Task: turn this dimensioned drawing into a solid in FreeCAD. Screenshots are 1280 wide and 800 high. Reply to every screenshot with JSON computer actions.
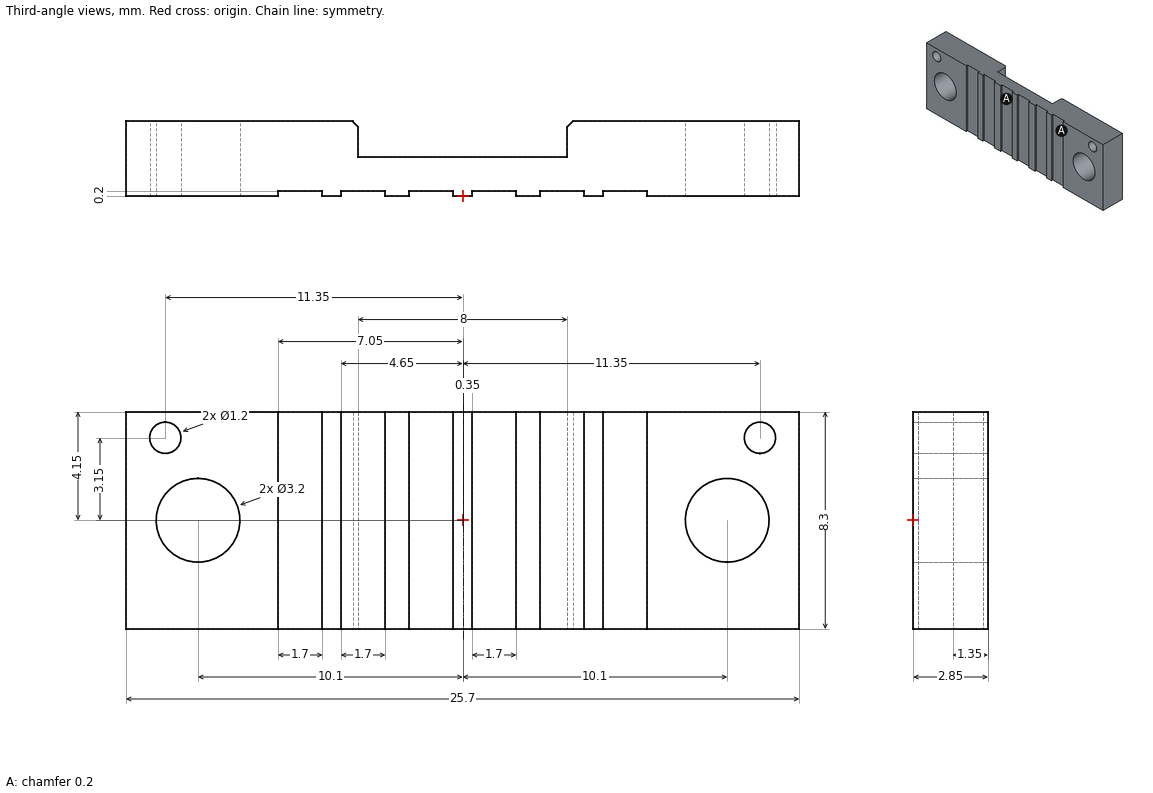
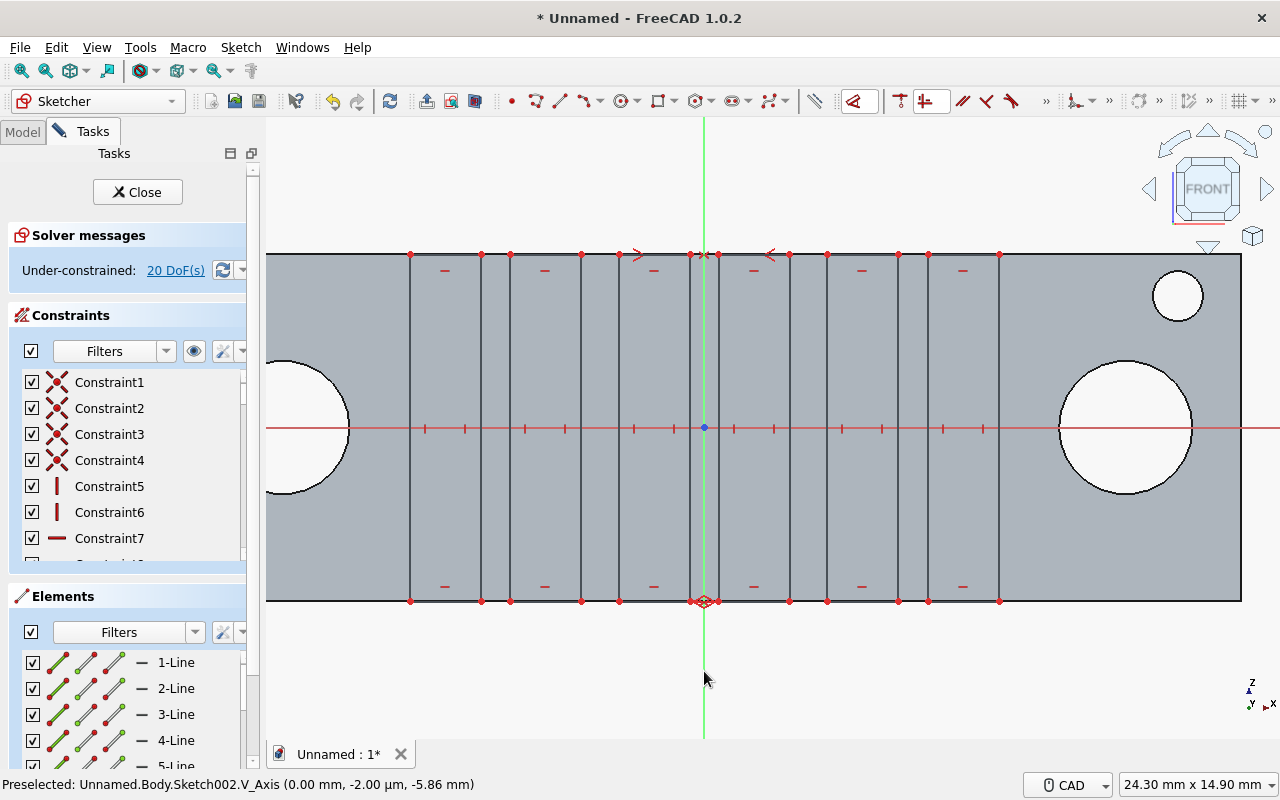
{"action": "left_click", "coordinate": [581, 255]}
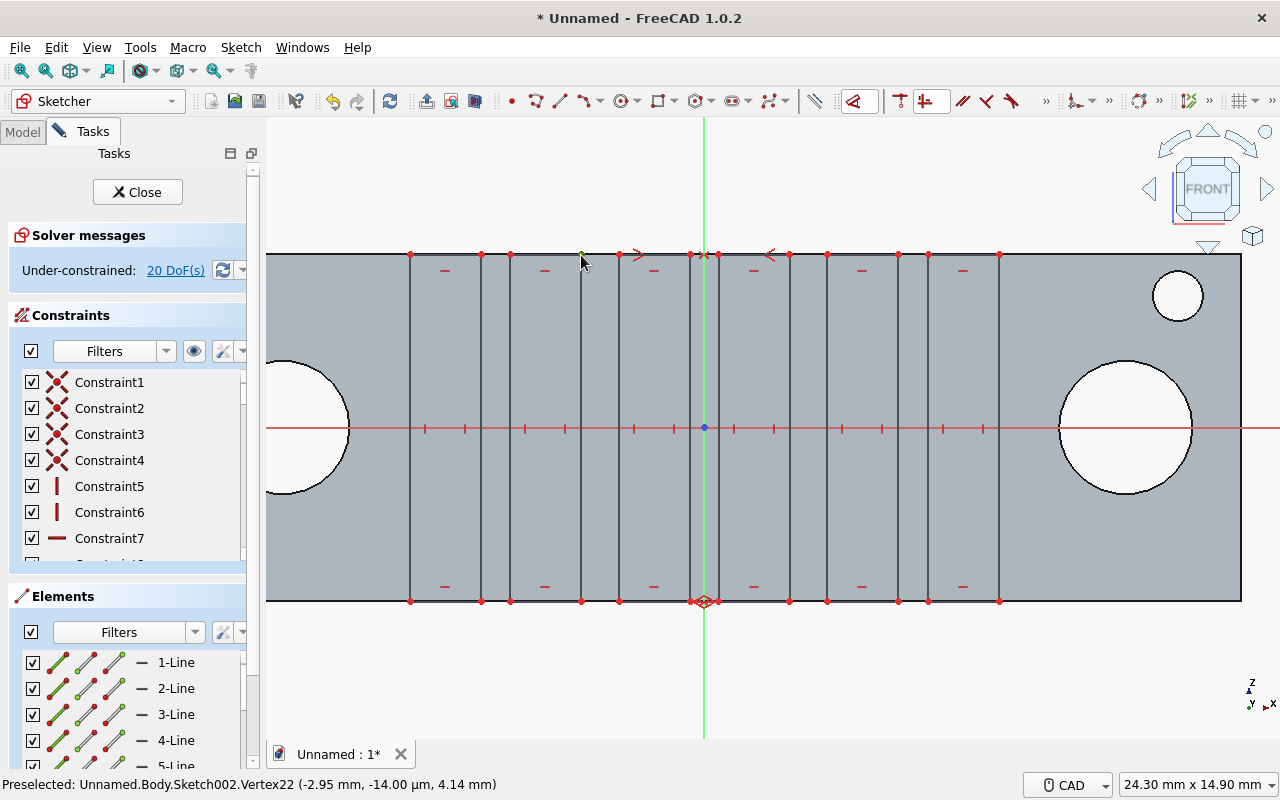
{"action": "left_click", "coordinate": [827, 255]}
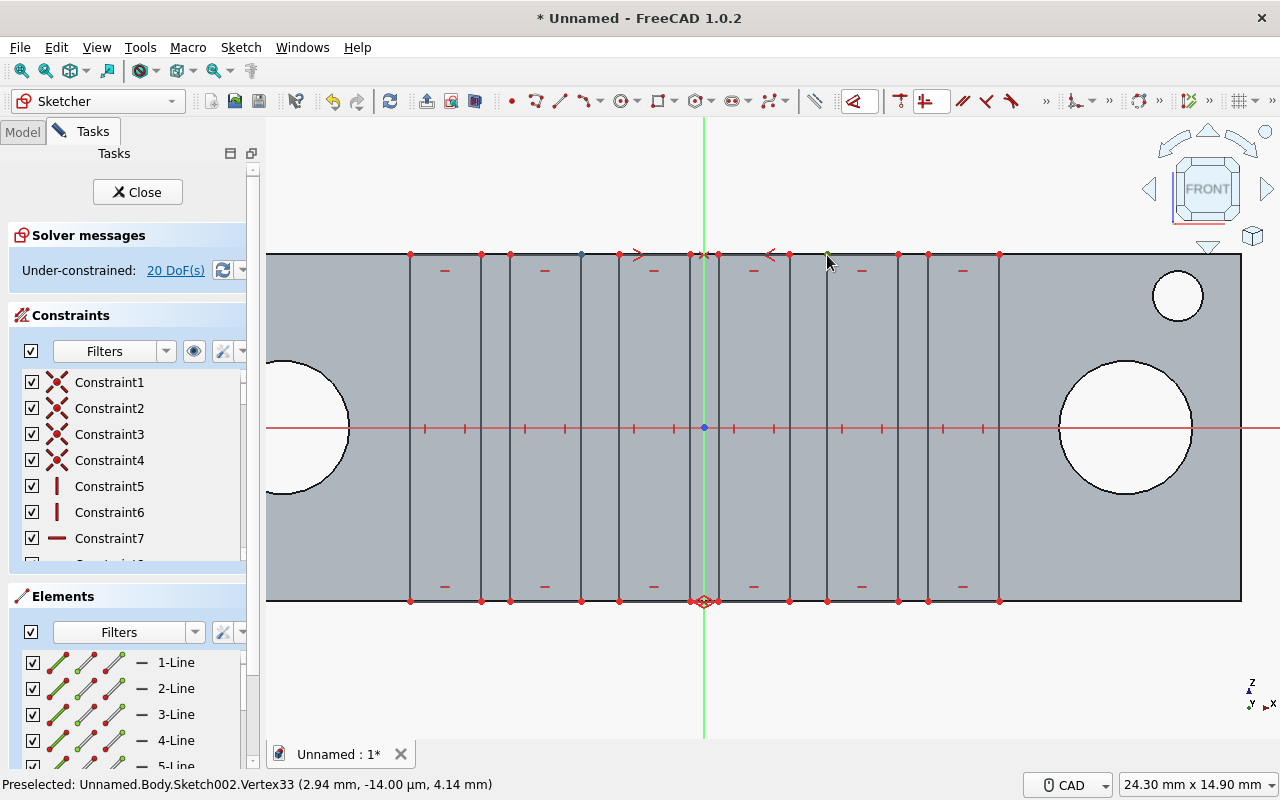
{"action": "left_click", "coordinate": [704, 671]}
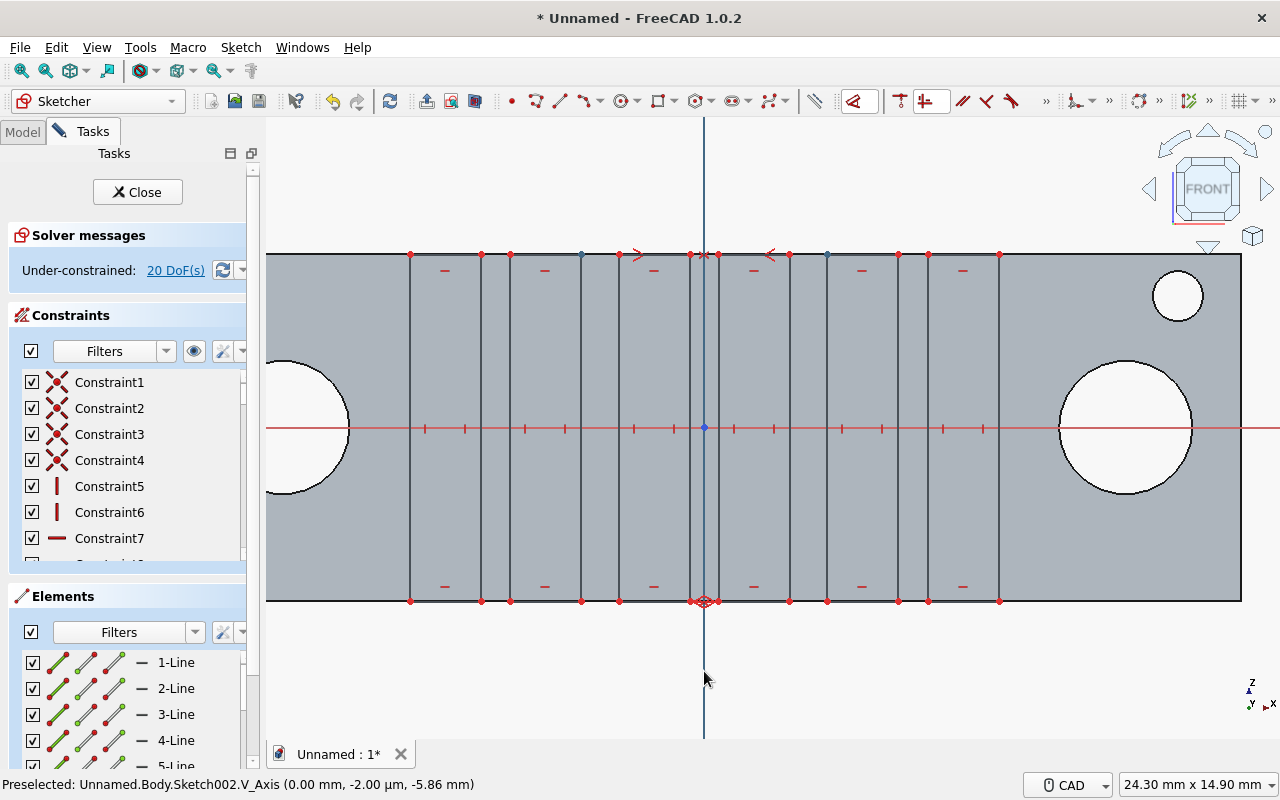
{"action": "key", "text": "s"}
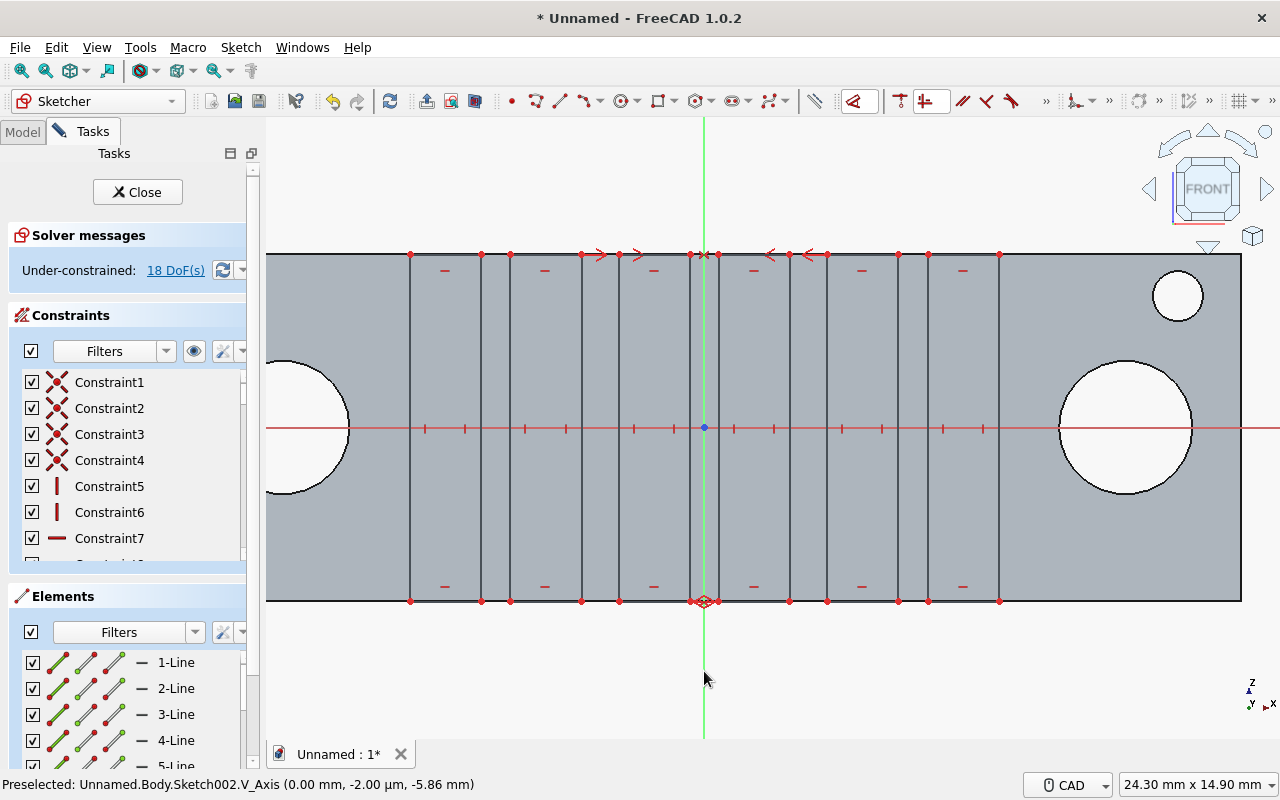
{"action": "left_click", "coordinate": [510, 602]}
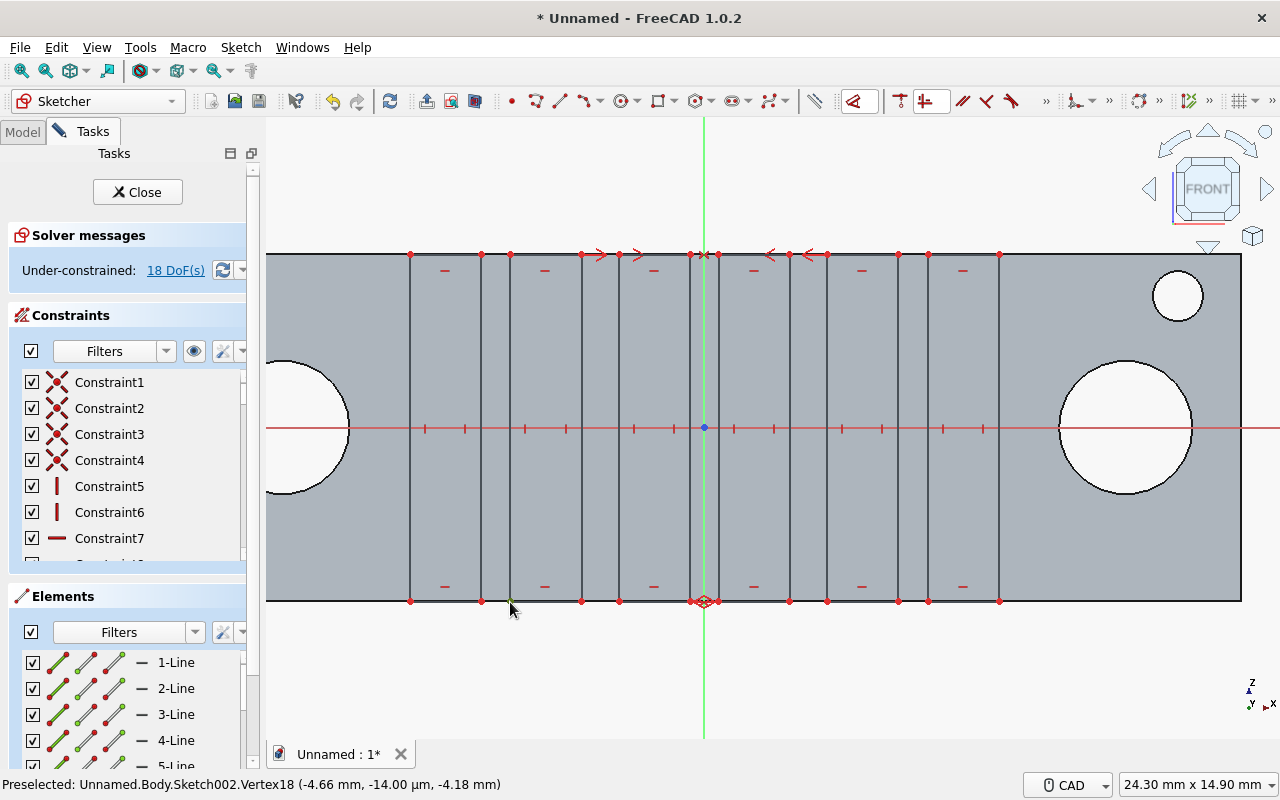
{"action": "left_click", "coordinate": [898, 602]}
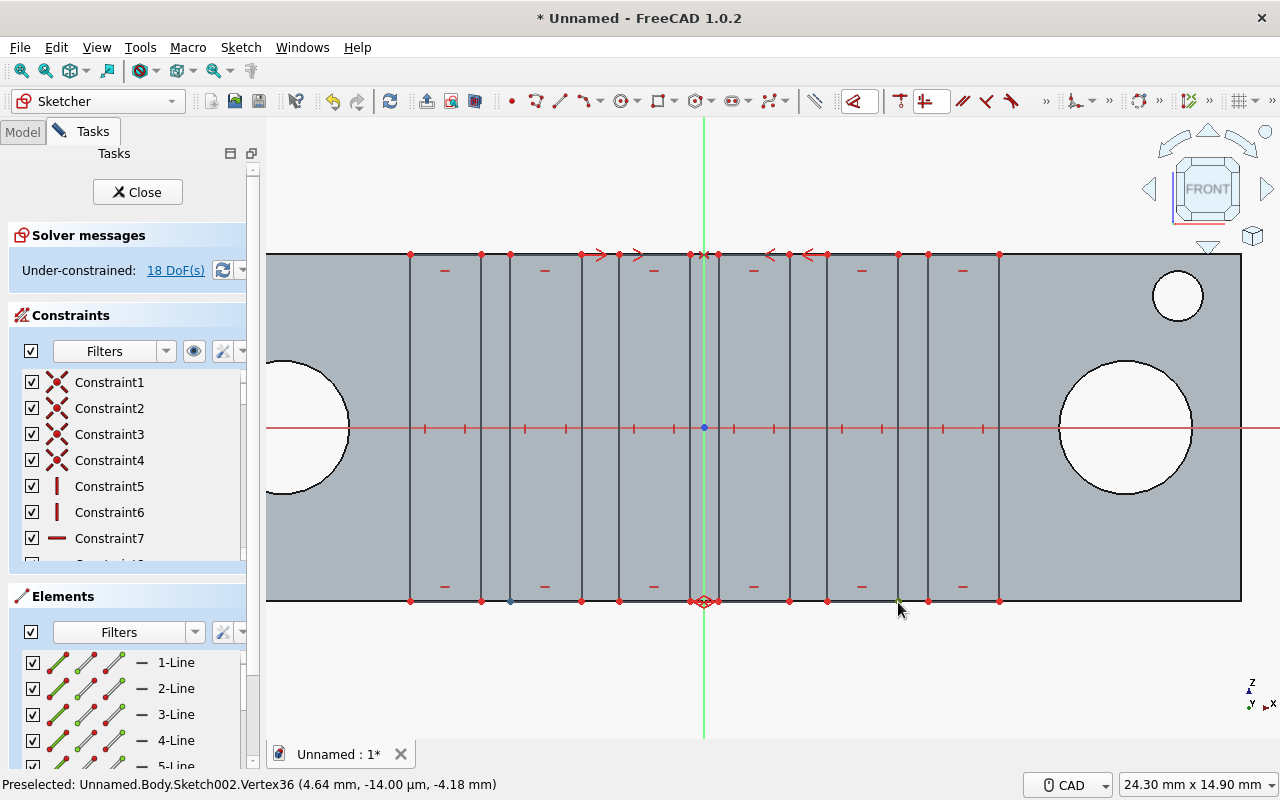
{"action": "left_click", "coordinate": [704, 671]}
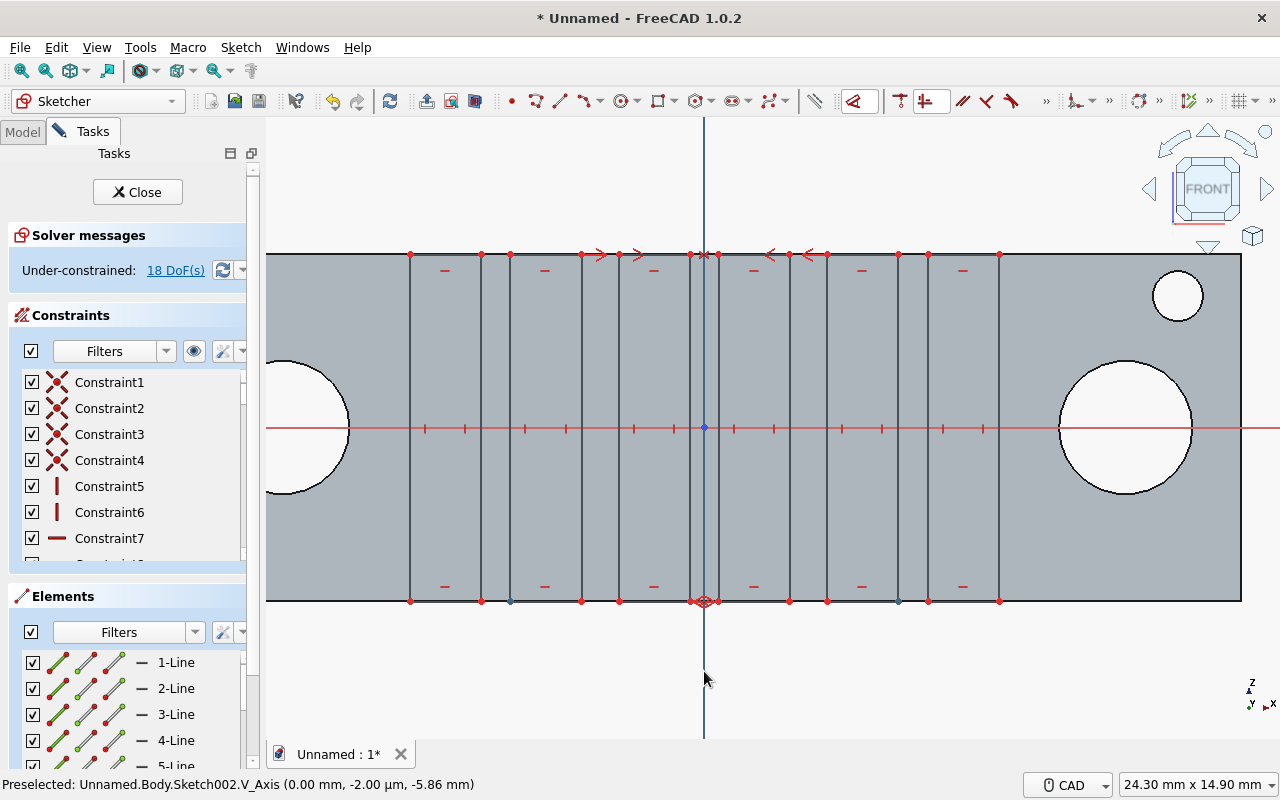
{"action": "key", "text": "s"}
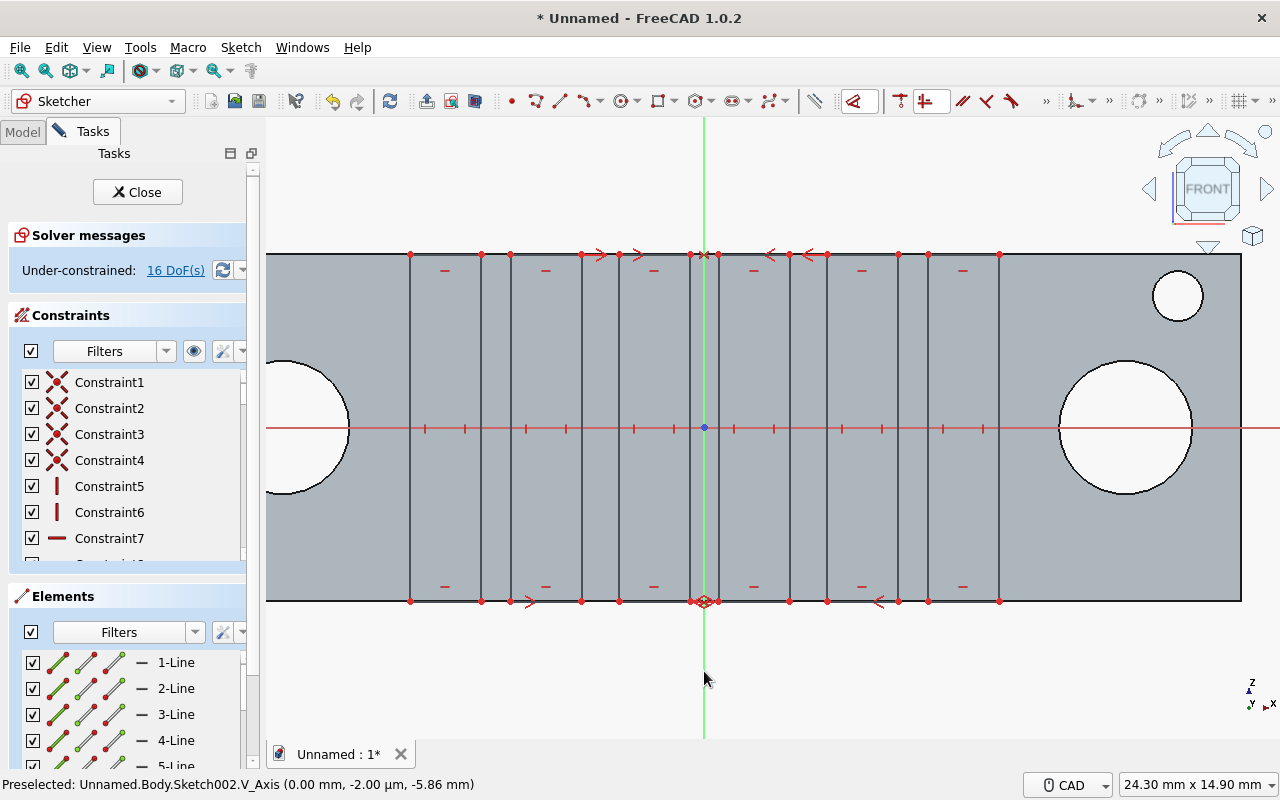
{"action": "left_click", "coordinate": [481, 255]}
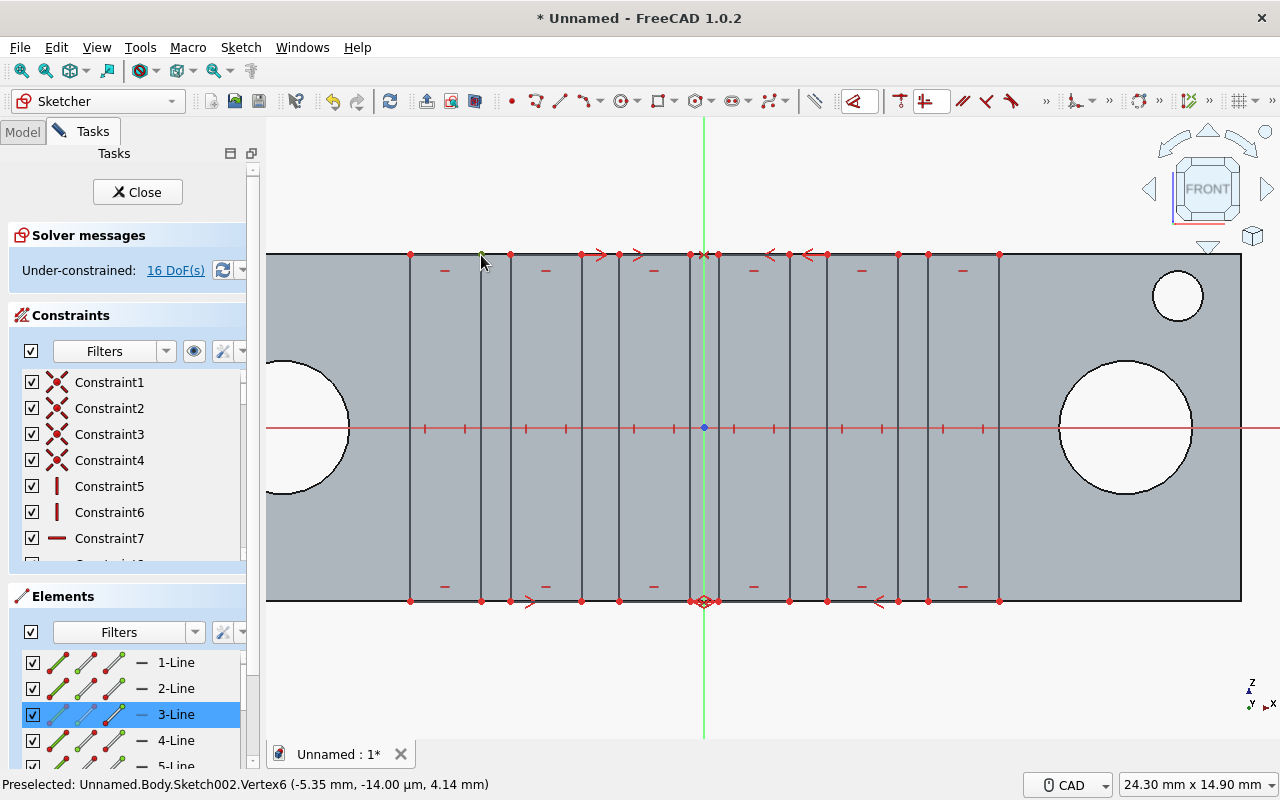
{"action": "left_click", "coordinate": [928, 255]}